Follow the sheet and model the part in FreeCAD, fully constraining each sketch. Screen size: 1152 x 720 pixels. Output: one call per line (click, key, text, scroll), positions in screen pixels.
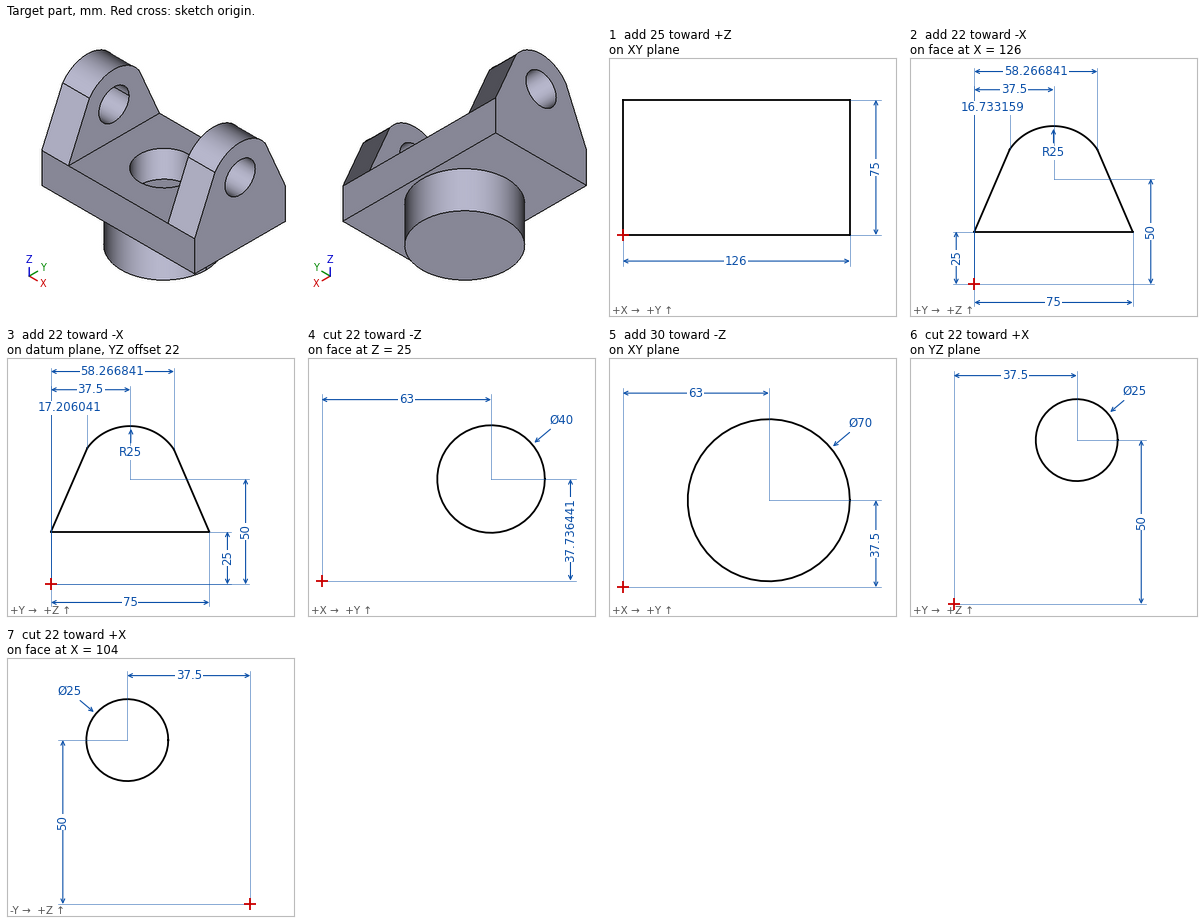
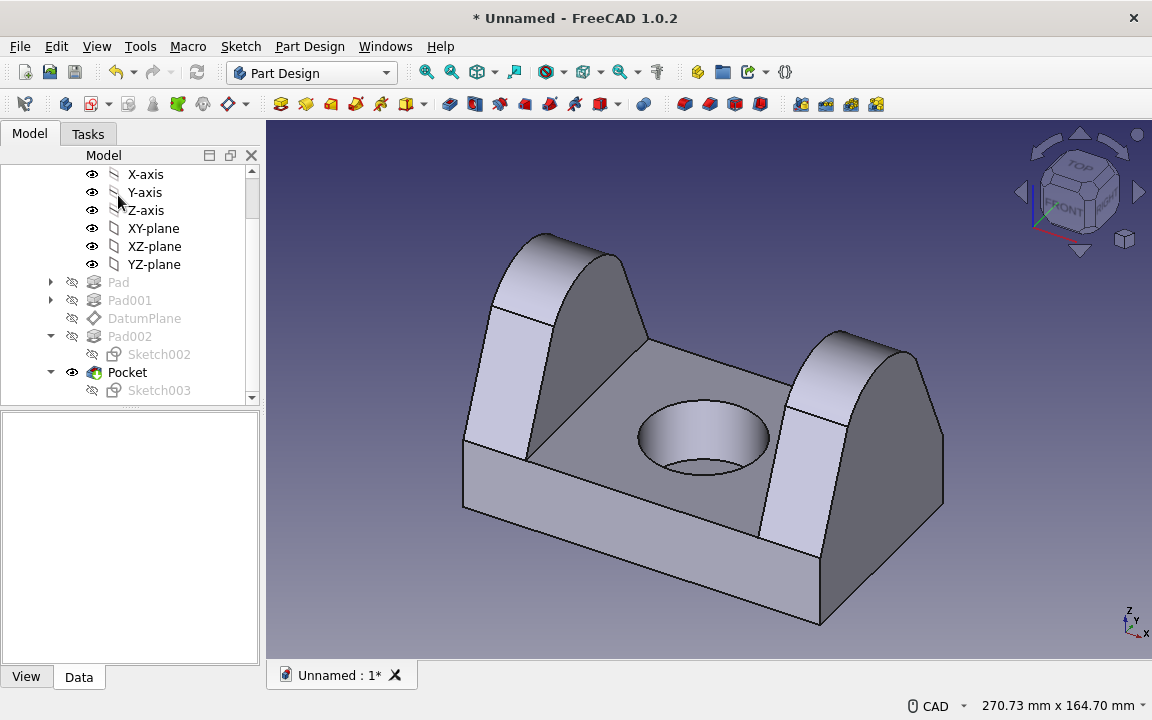
click(90, 104)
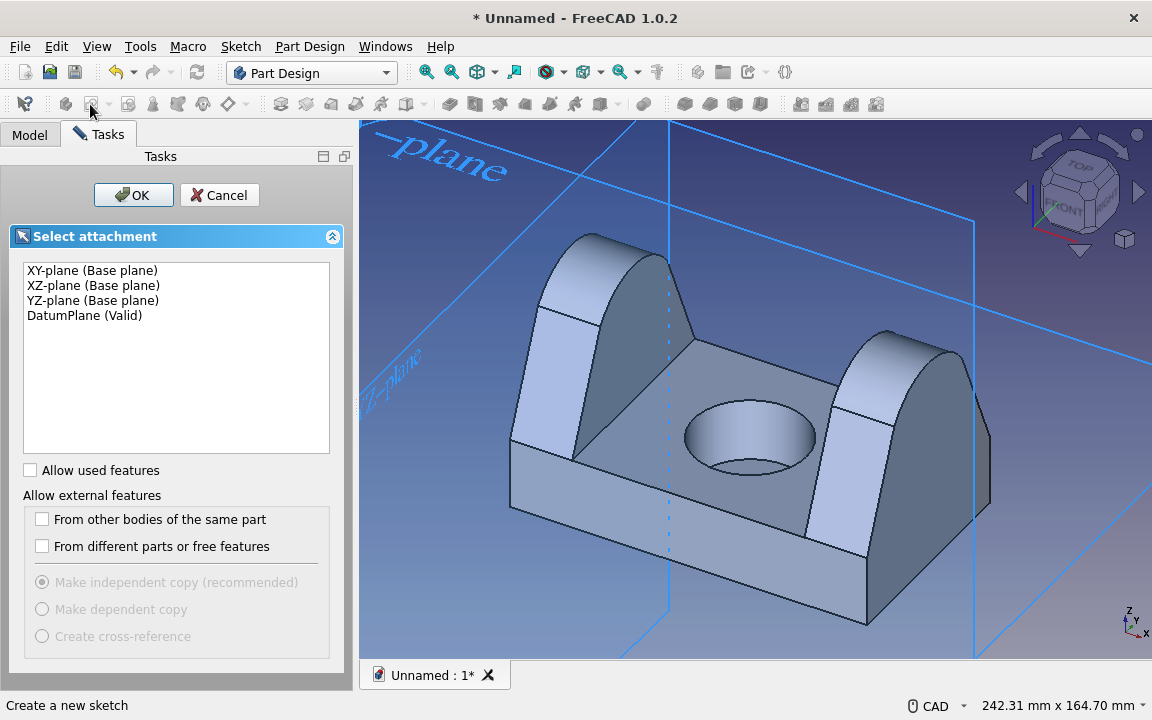
click(84, 270)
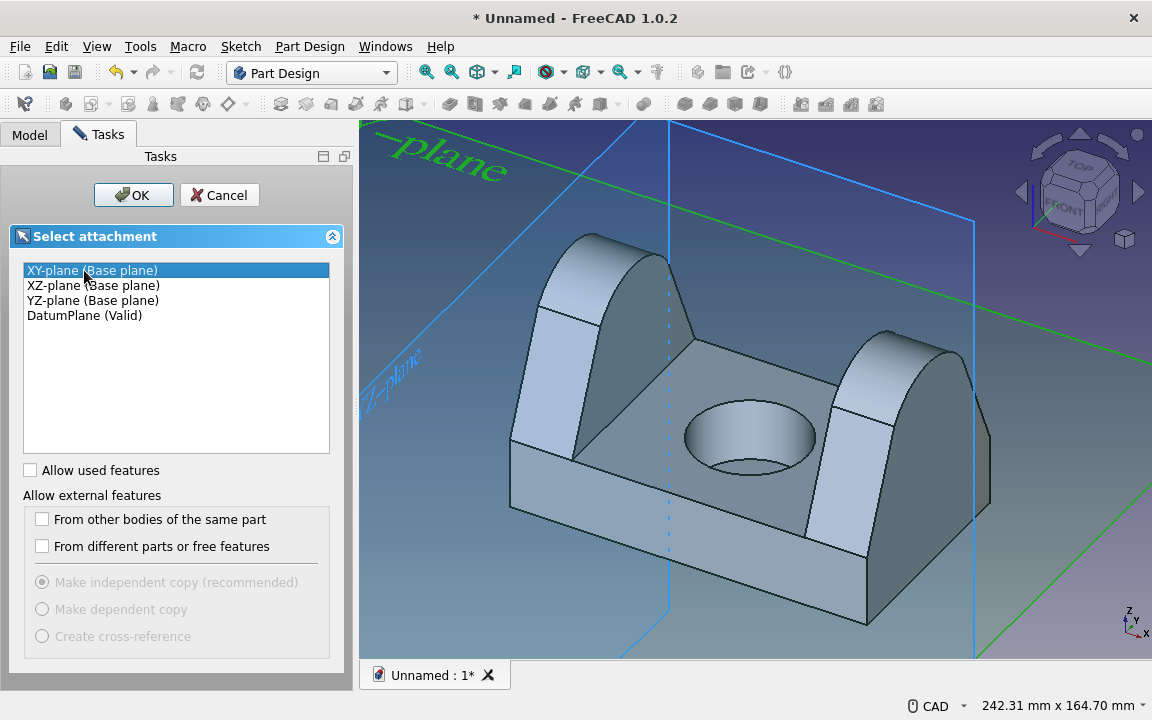
click(134, 195)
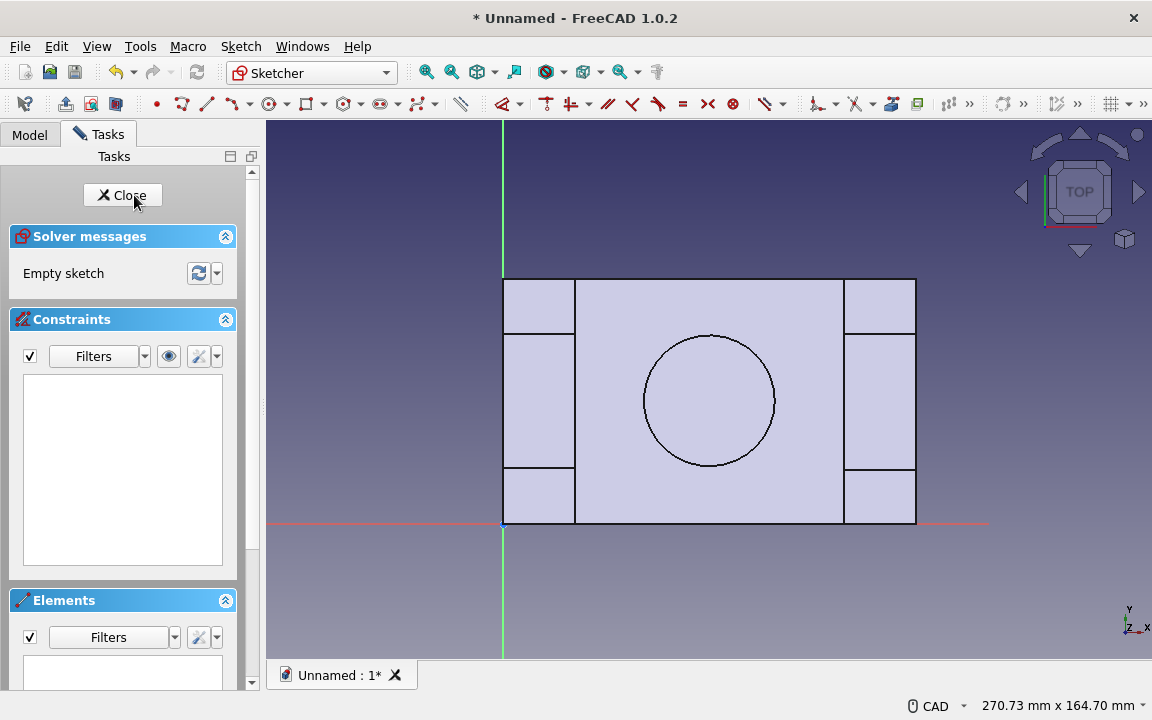
click(116, 104)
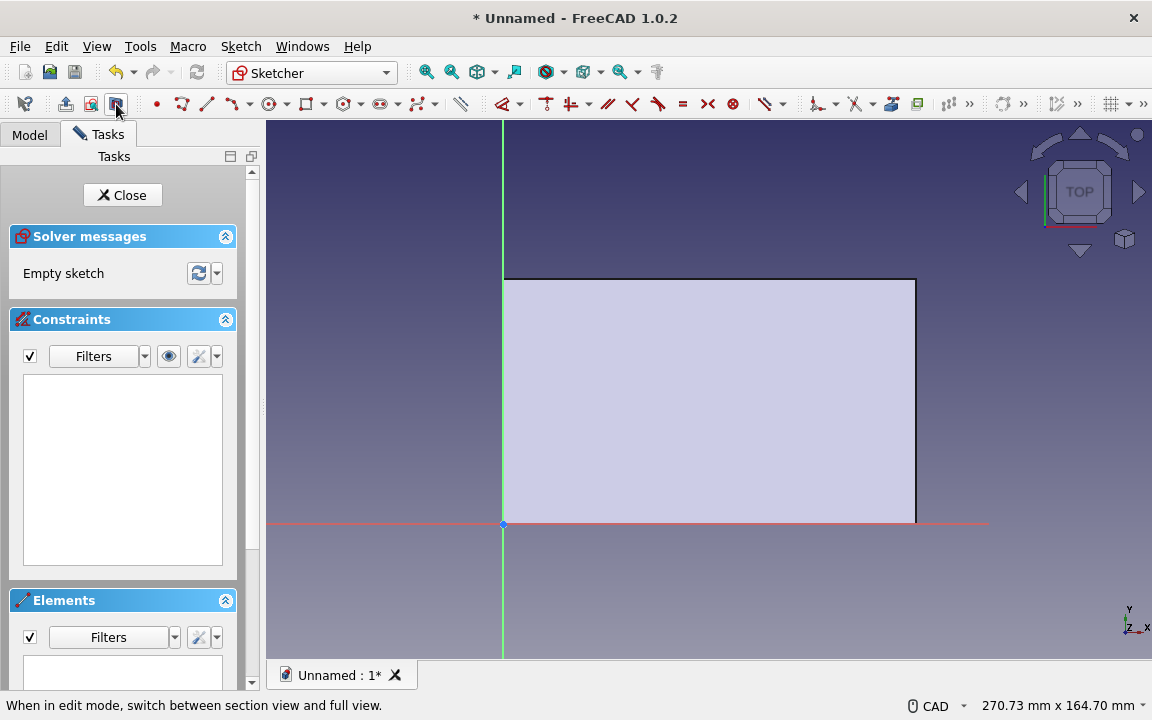
scroll(710, 438, up, 2)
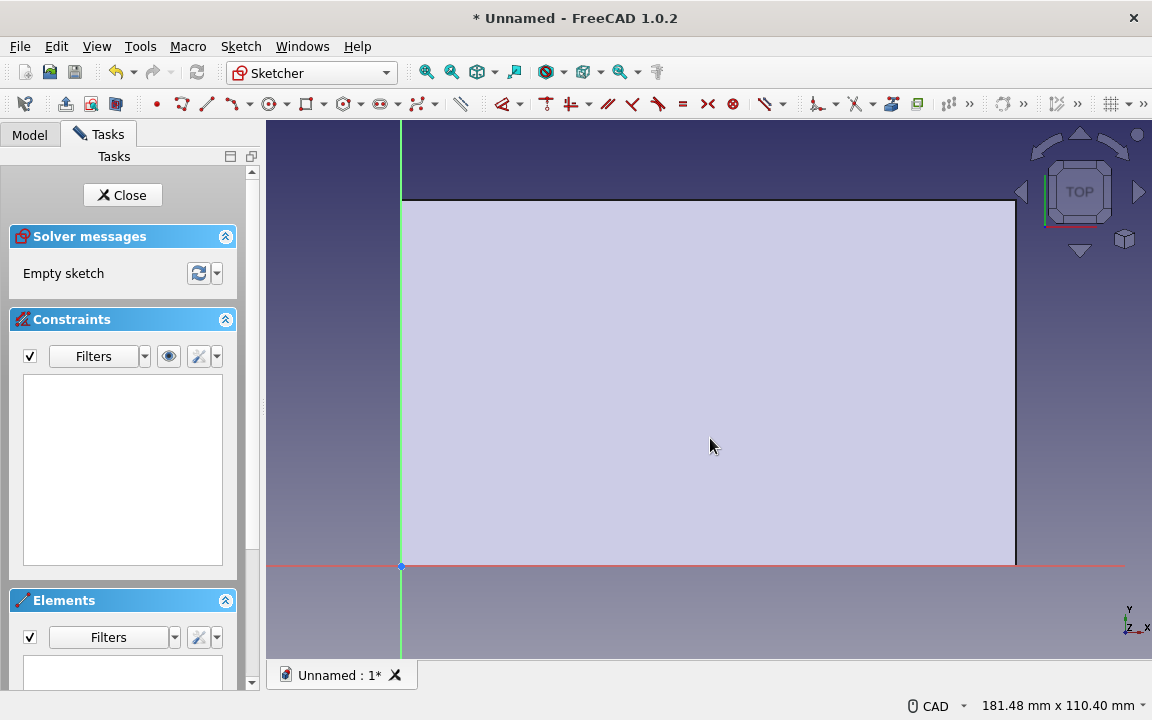
click(268, 104)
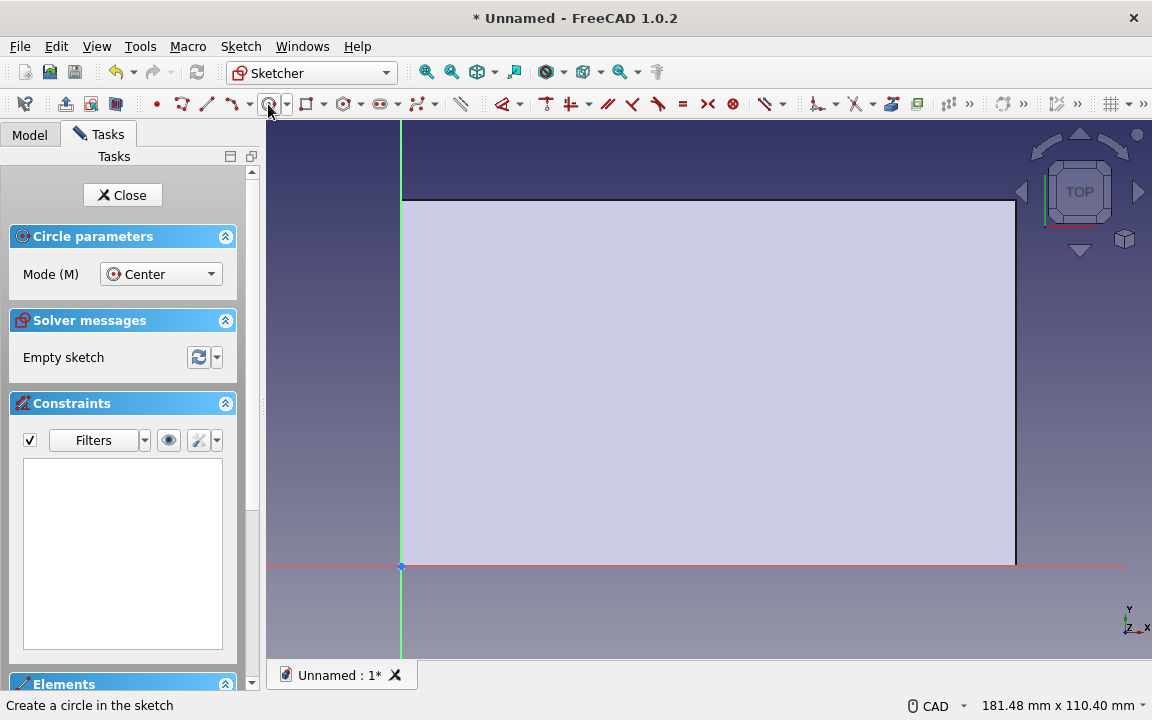
click(709, 383)
move(830, 263)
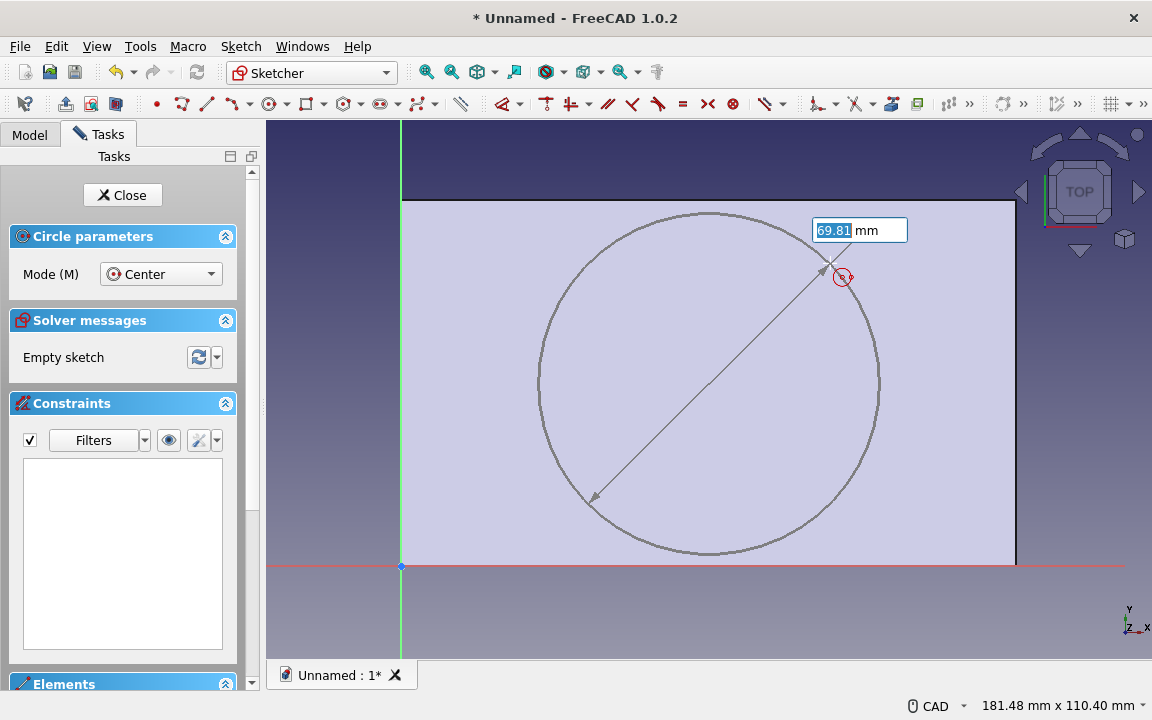
text(70)
key(Return)
key(Escape)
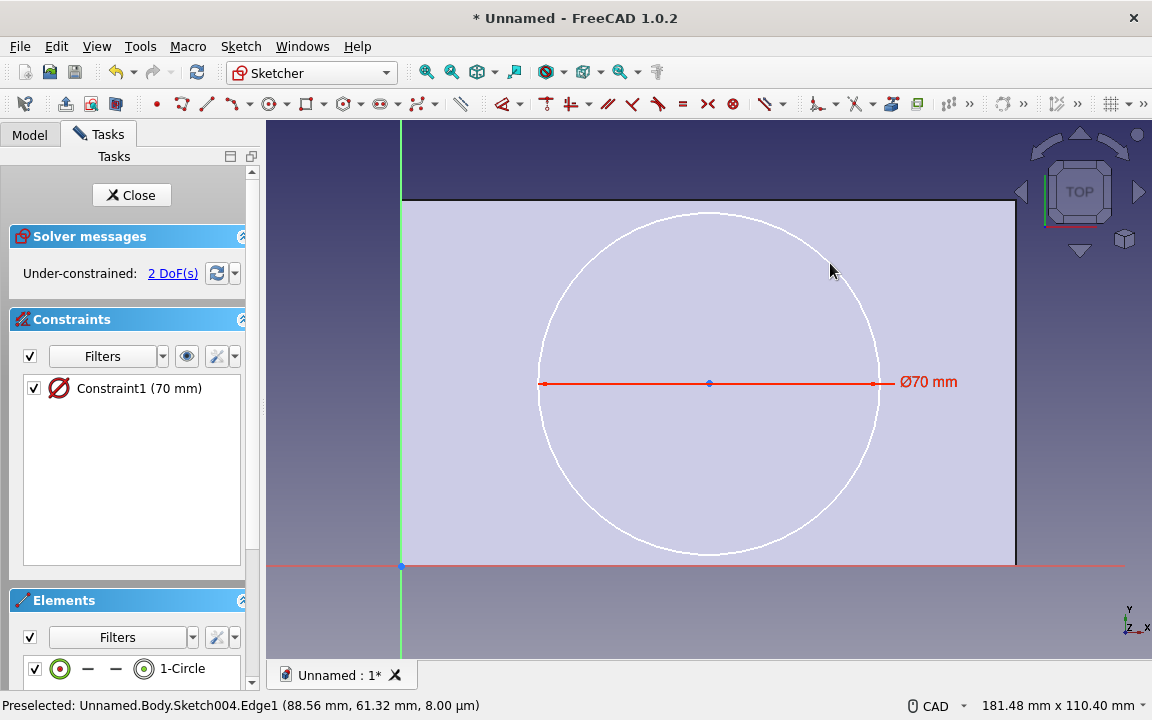
click(502, 104)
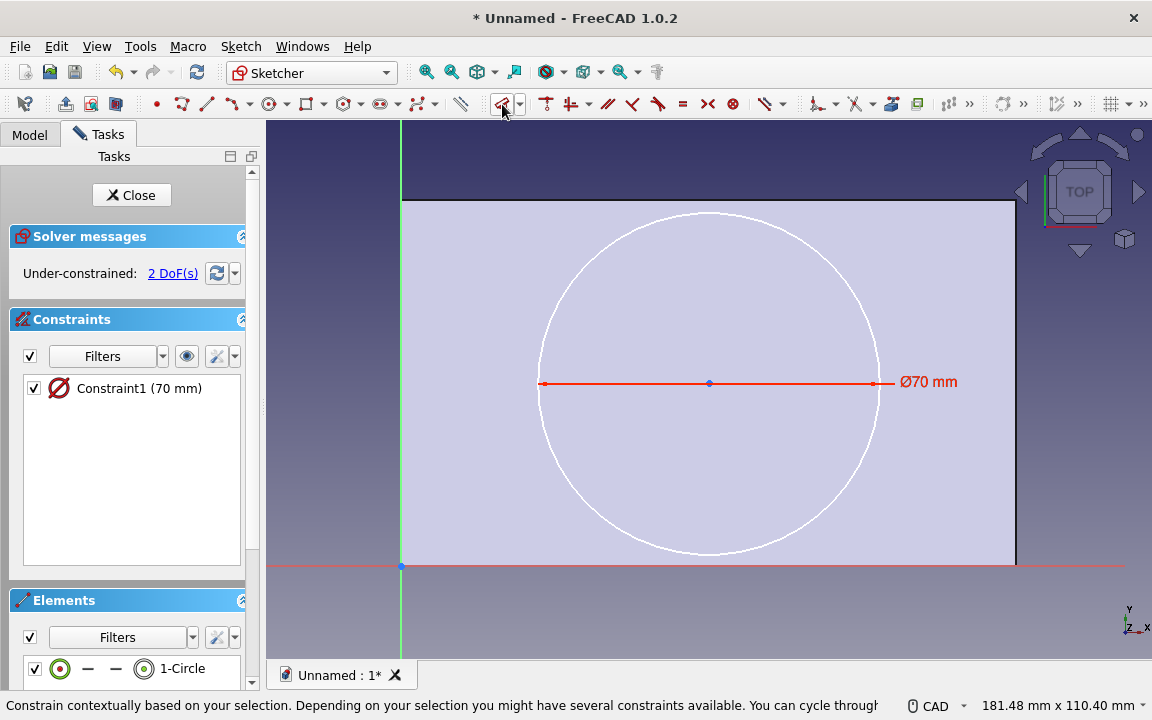
click(709, 384)
click(555, 600)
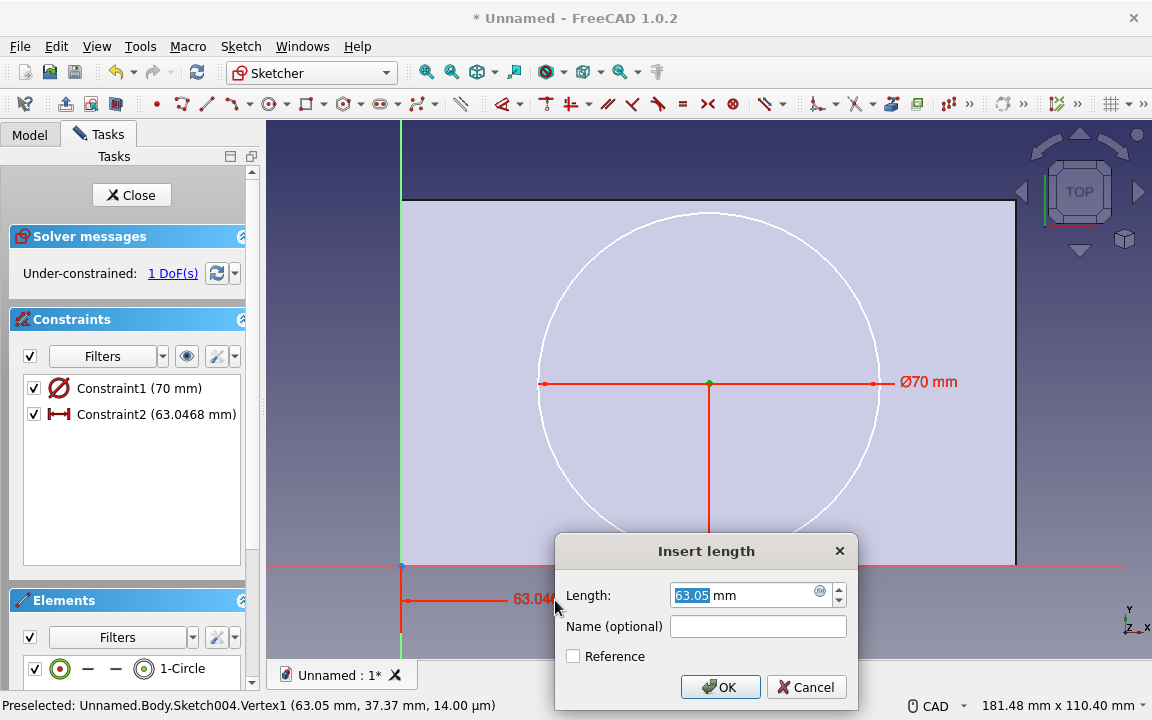
text(63)
key(Return)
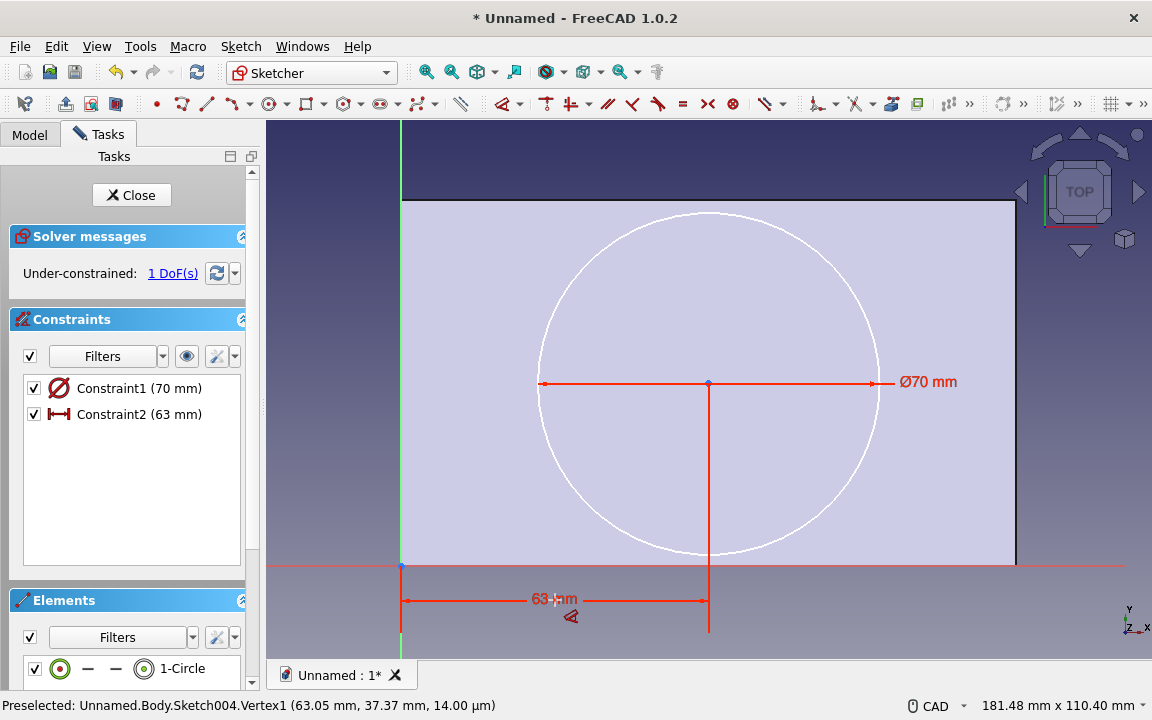
click(709, 384)
click(367, 475)